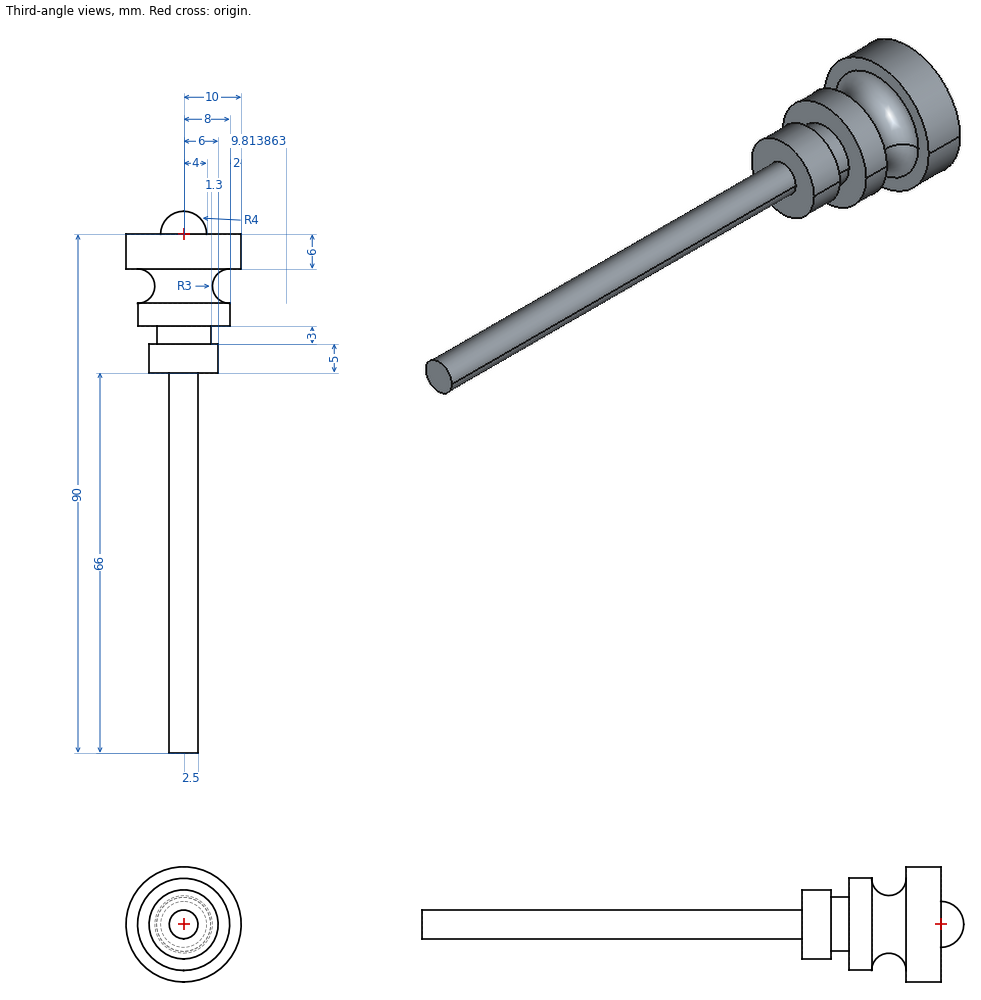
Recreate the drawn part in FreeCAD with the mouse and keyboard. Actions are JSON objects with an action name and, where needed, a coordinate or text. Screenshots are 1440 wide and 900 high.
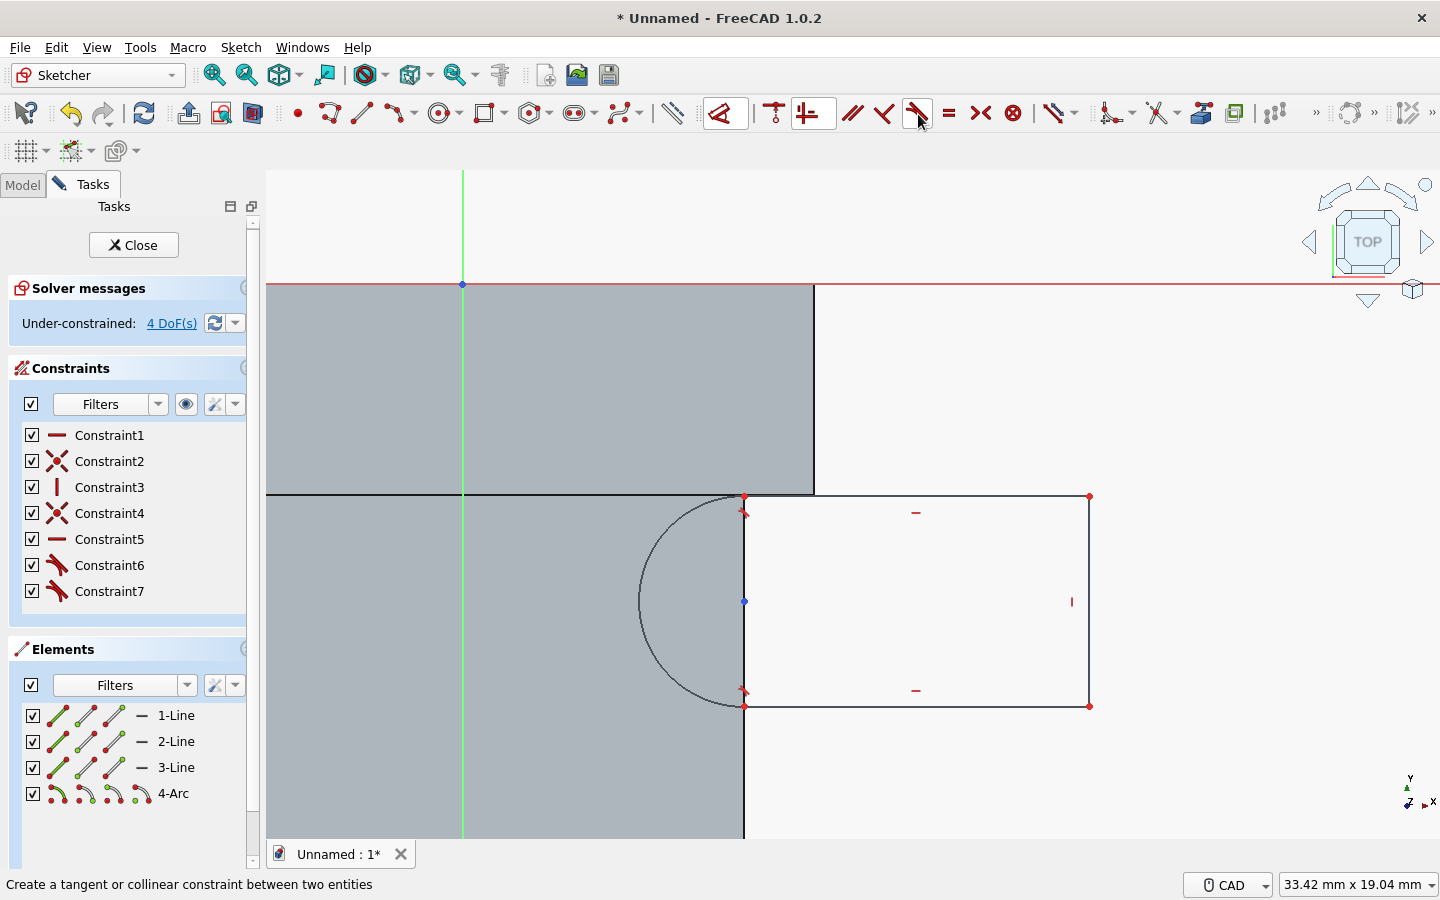
{"action": "left_click", "coordinate": [659, 539]}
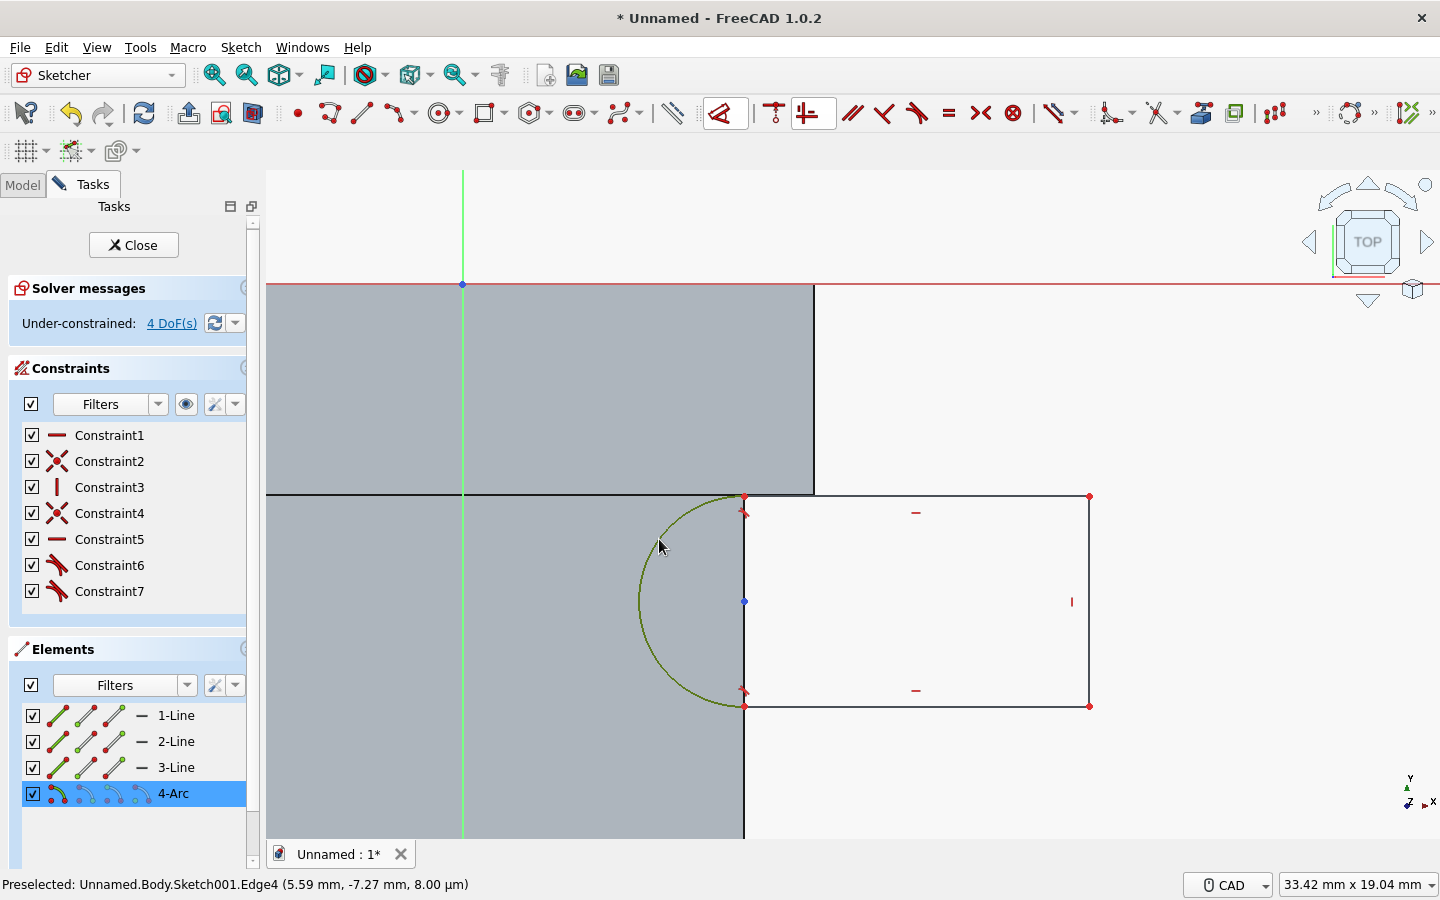
{"action": "key", "text": "k r"}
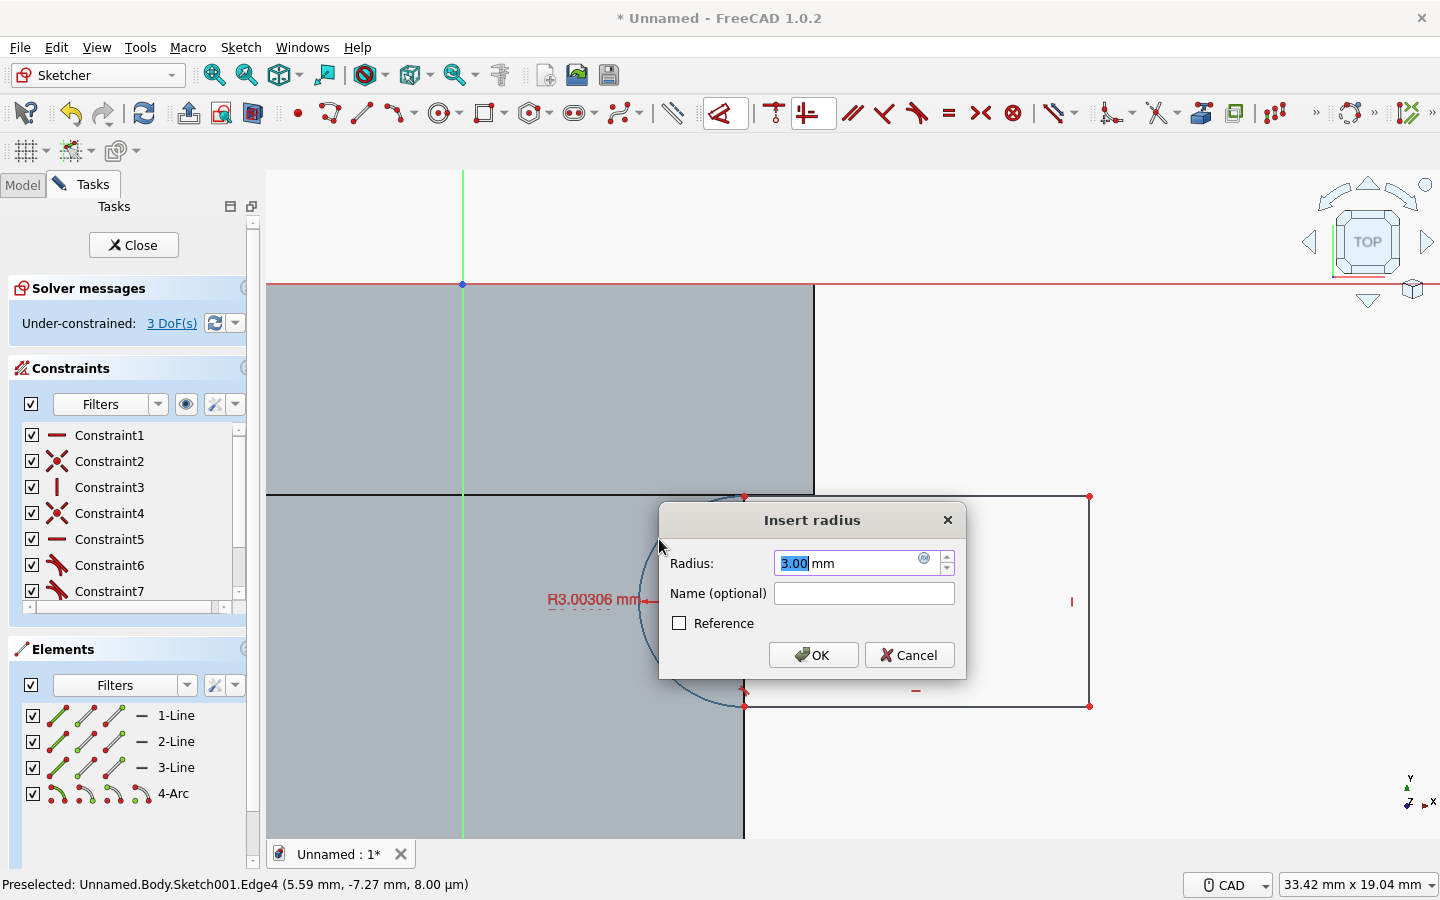
{"action": "type", "text": "3"}
{"action": "key", "text": "Return"}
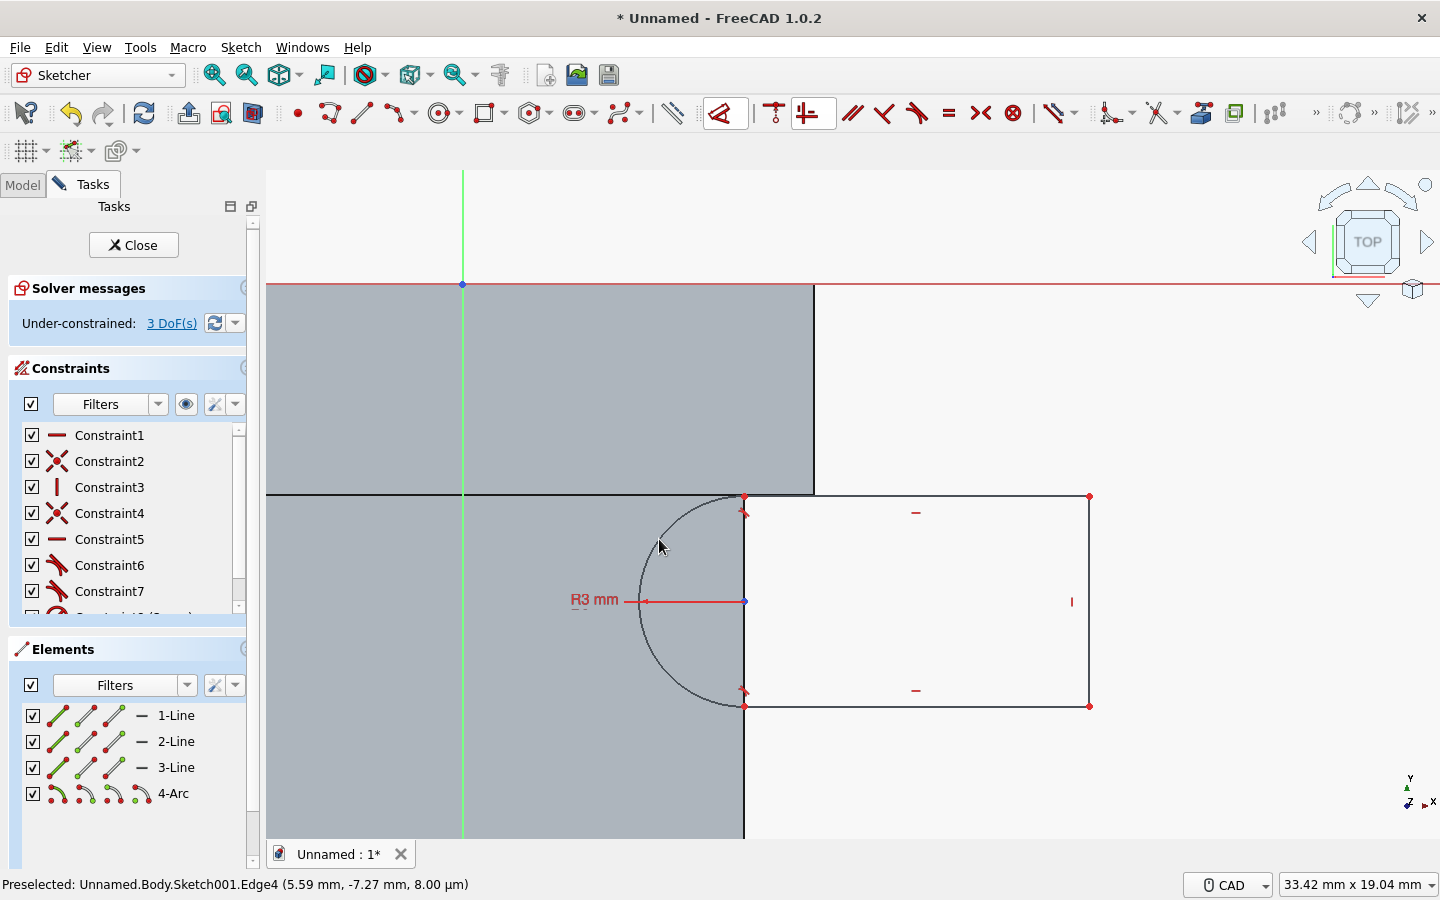
{"action": "left_click", "coordinate": [744, 707]}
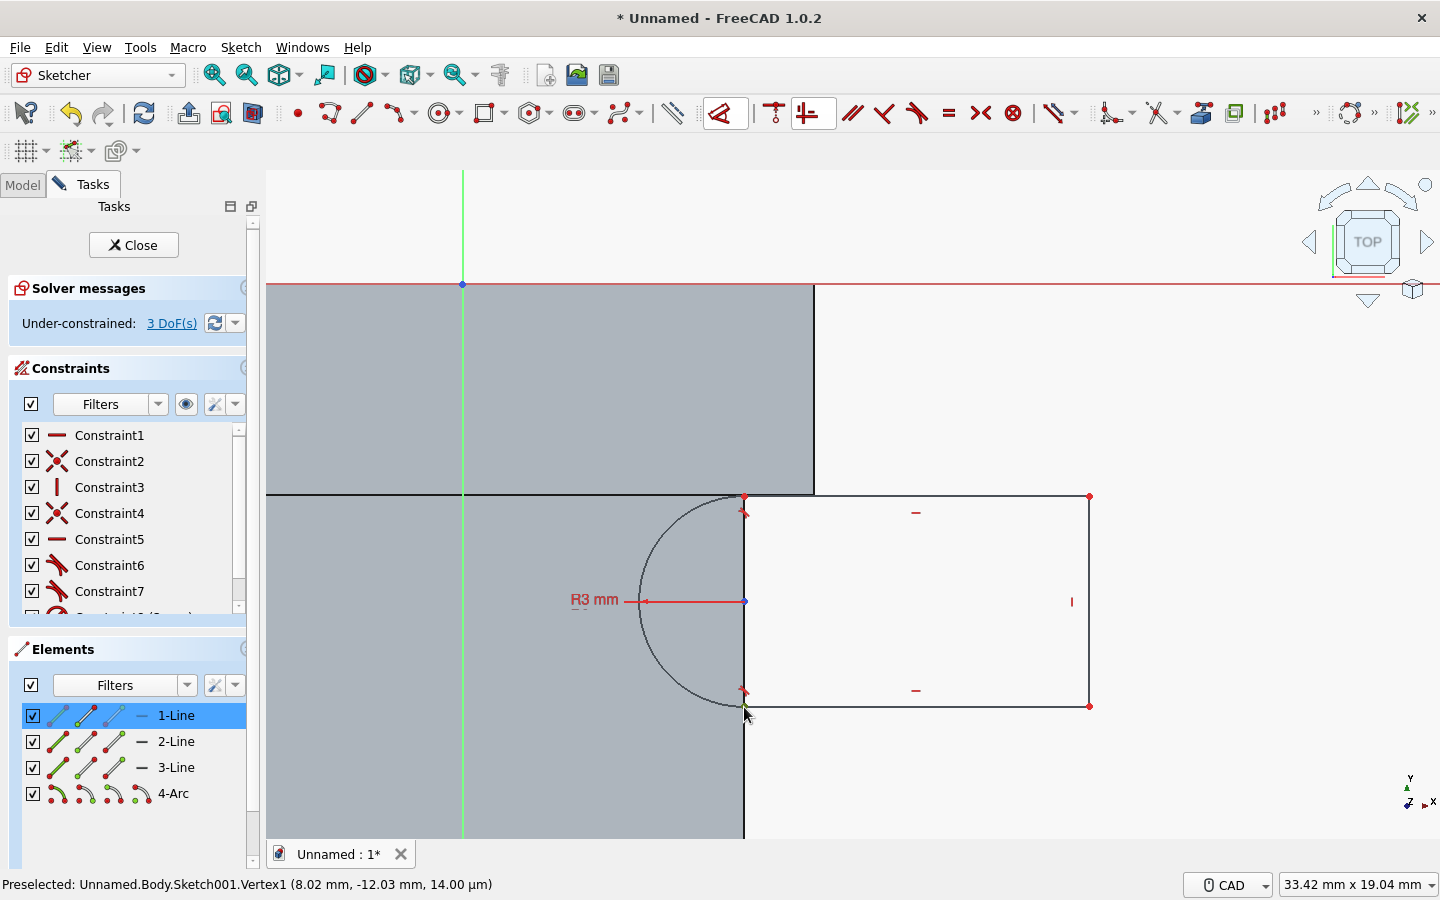
{"action": "key", "text": "l"}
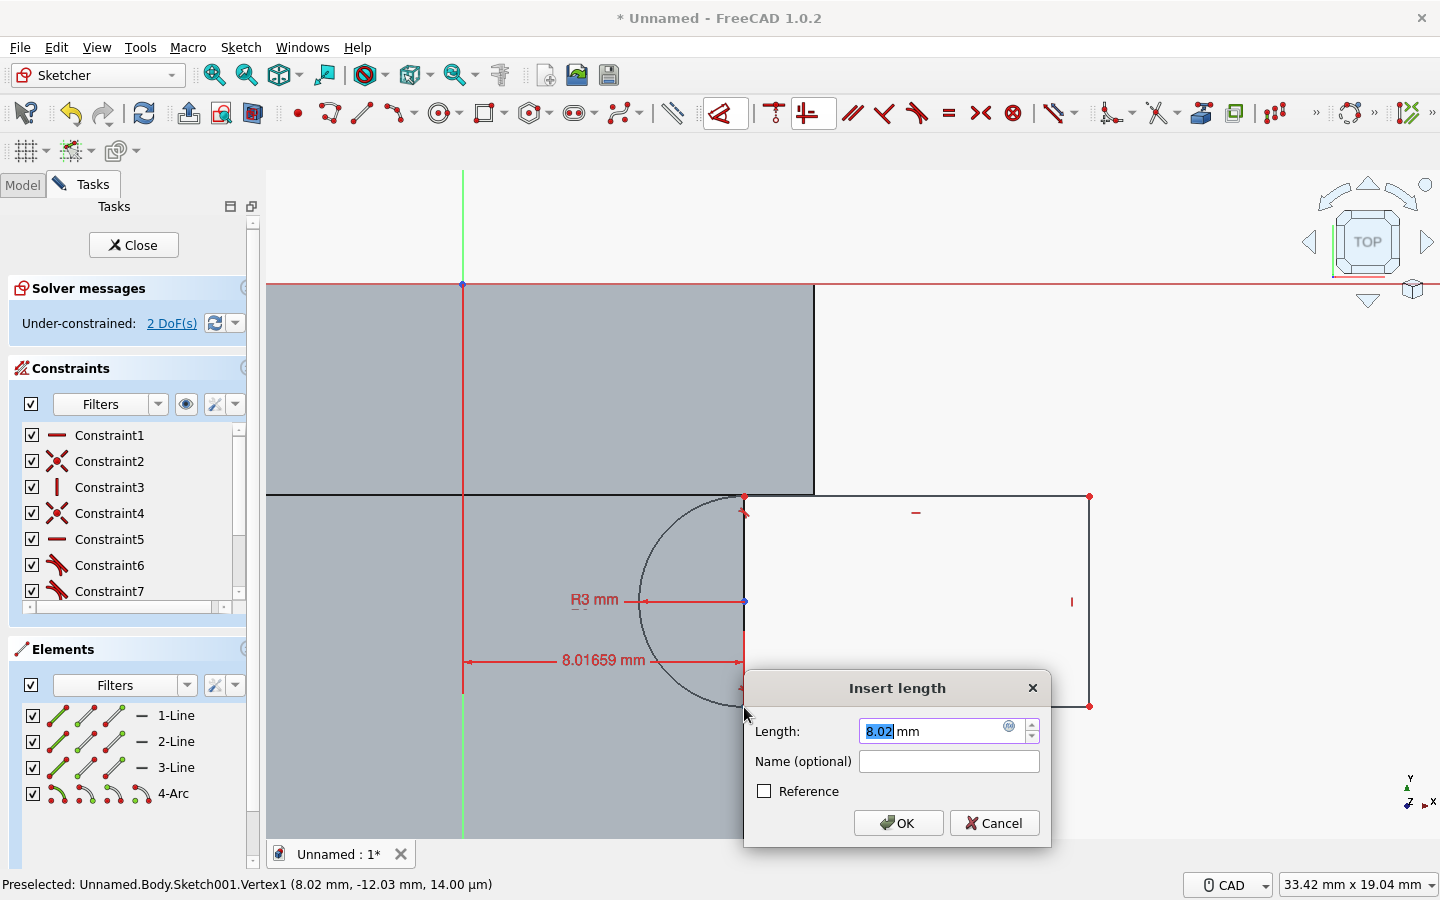
{"action": "type", "text": "8"}
{"action": "key", "text": "Return"}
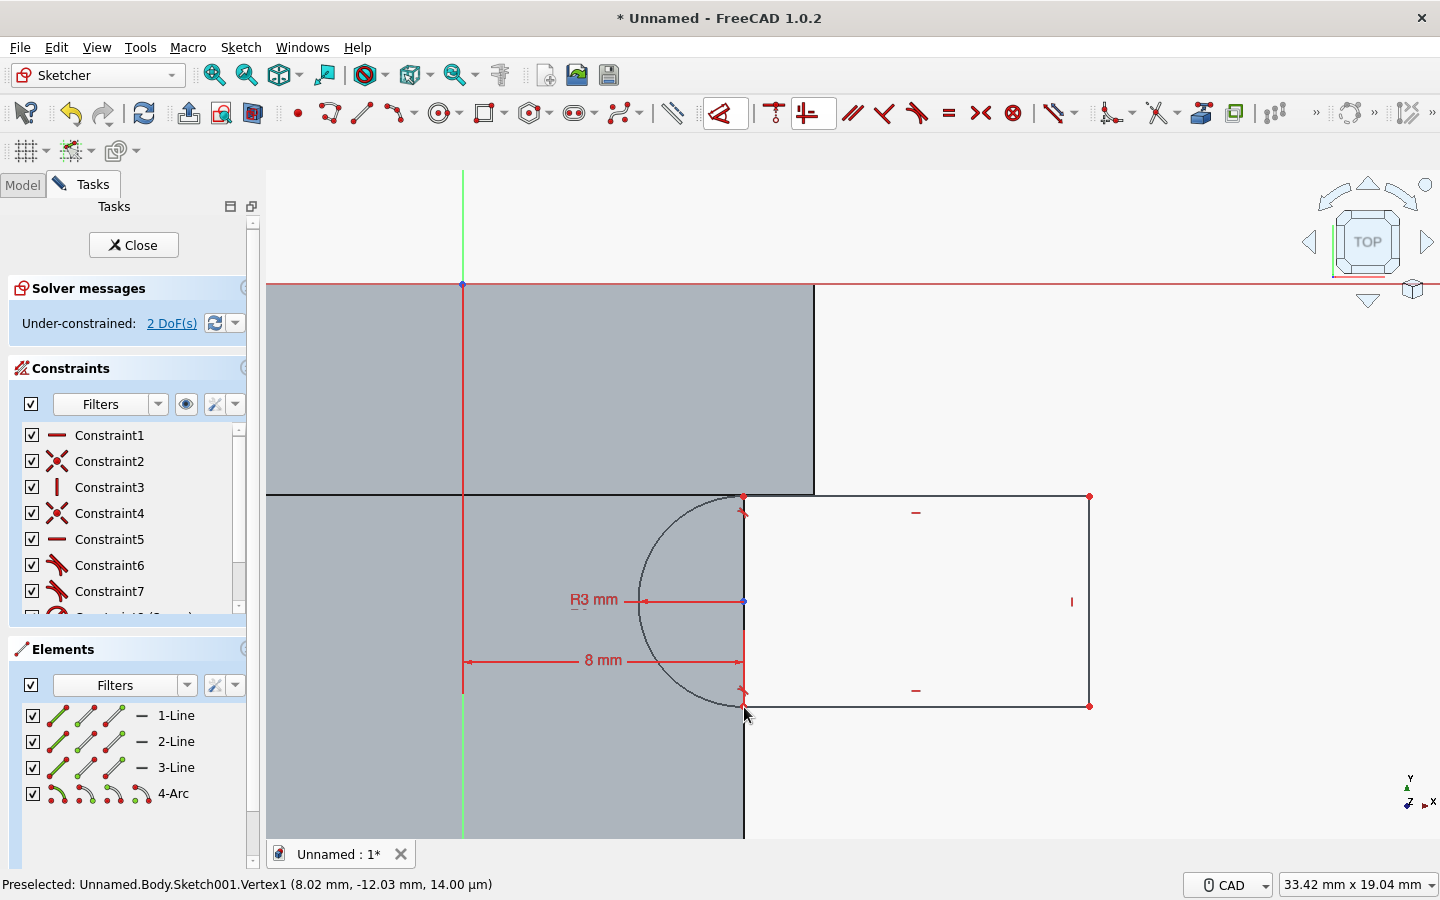
{"action": "left_click", "coordinate": [1089, 496]}